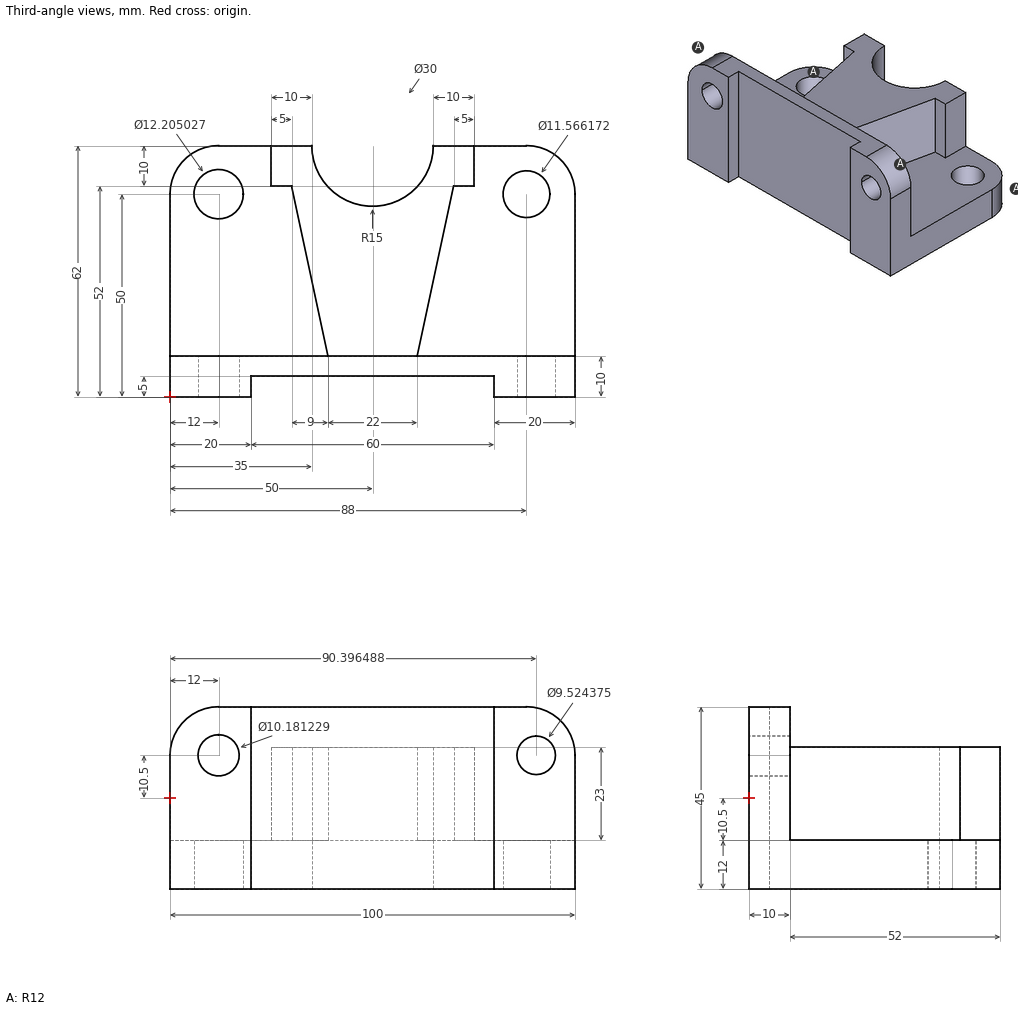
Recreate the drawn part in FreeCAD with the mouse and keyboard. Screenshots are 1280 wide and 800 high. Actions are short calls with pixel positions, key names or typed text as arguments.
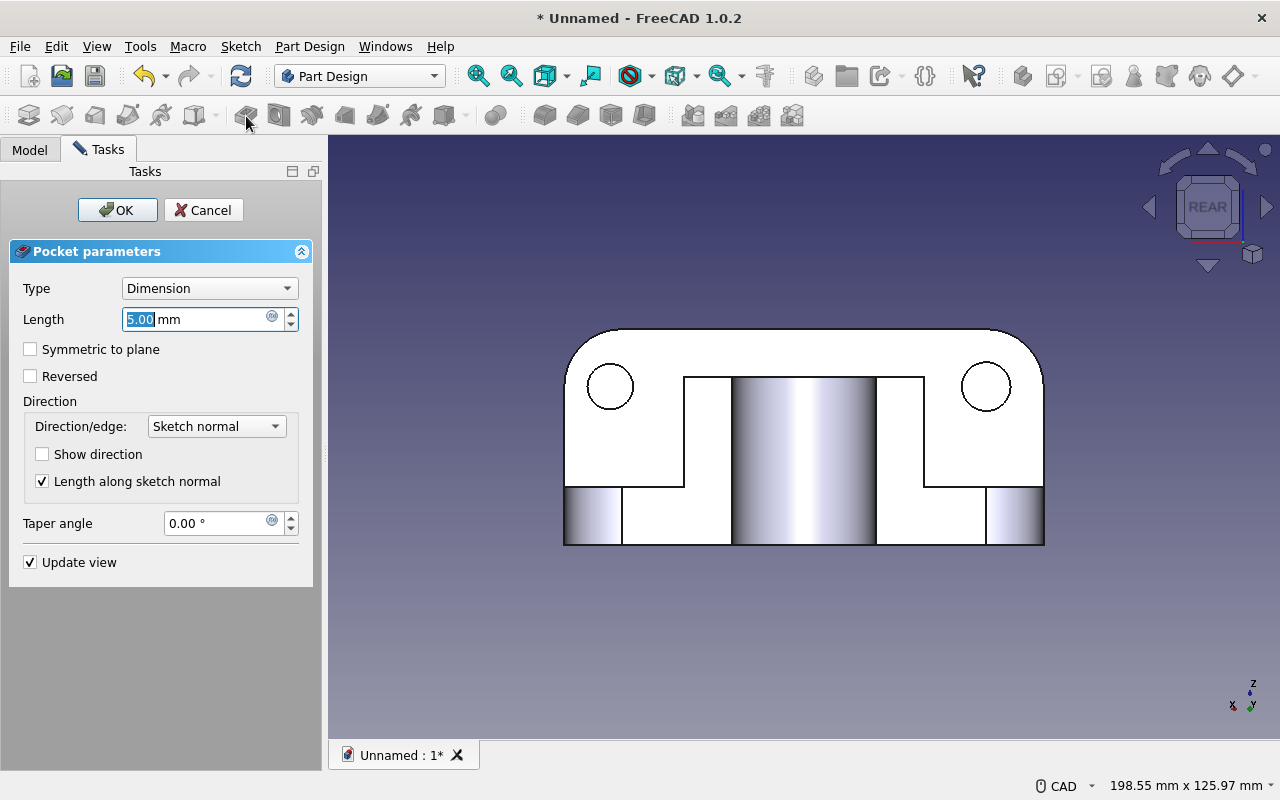
click(210, 288)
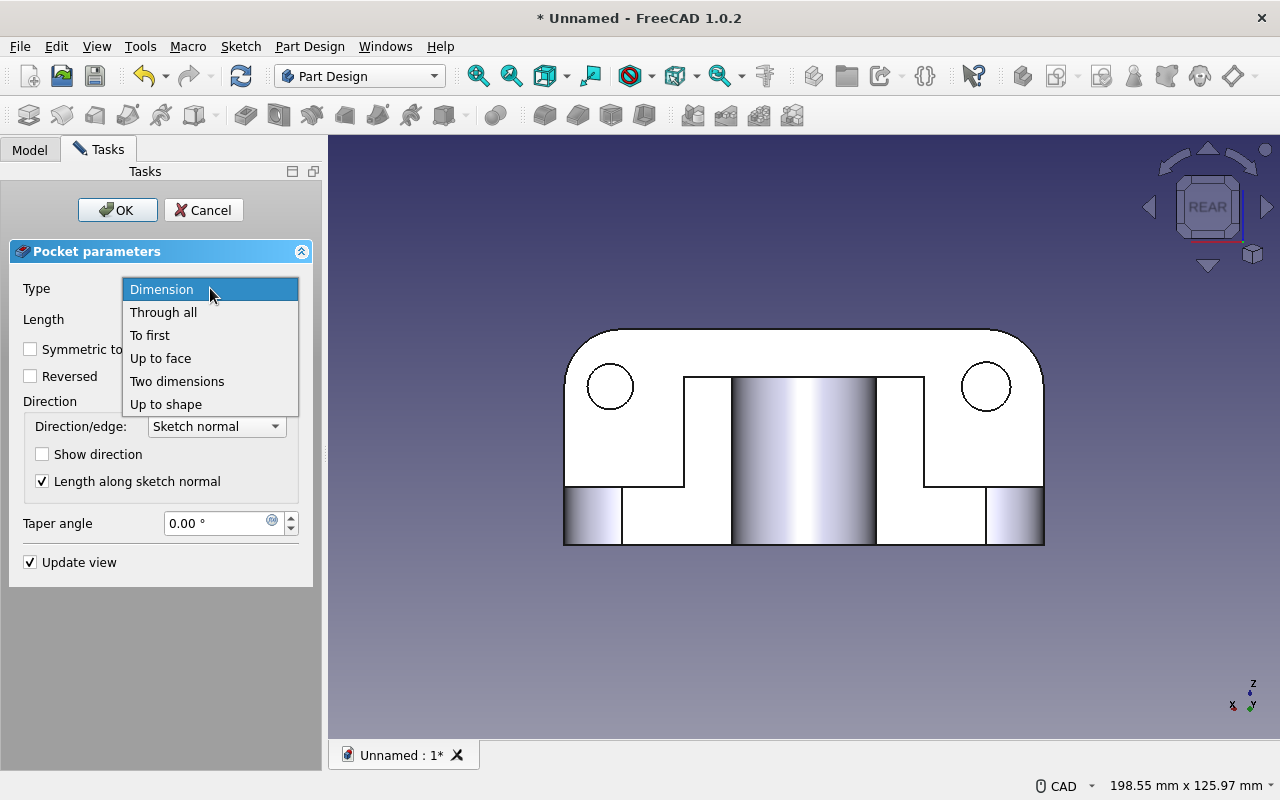
click(208, 312)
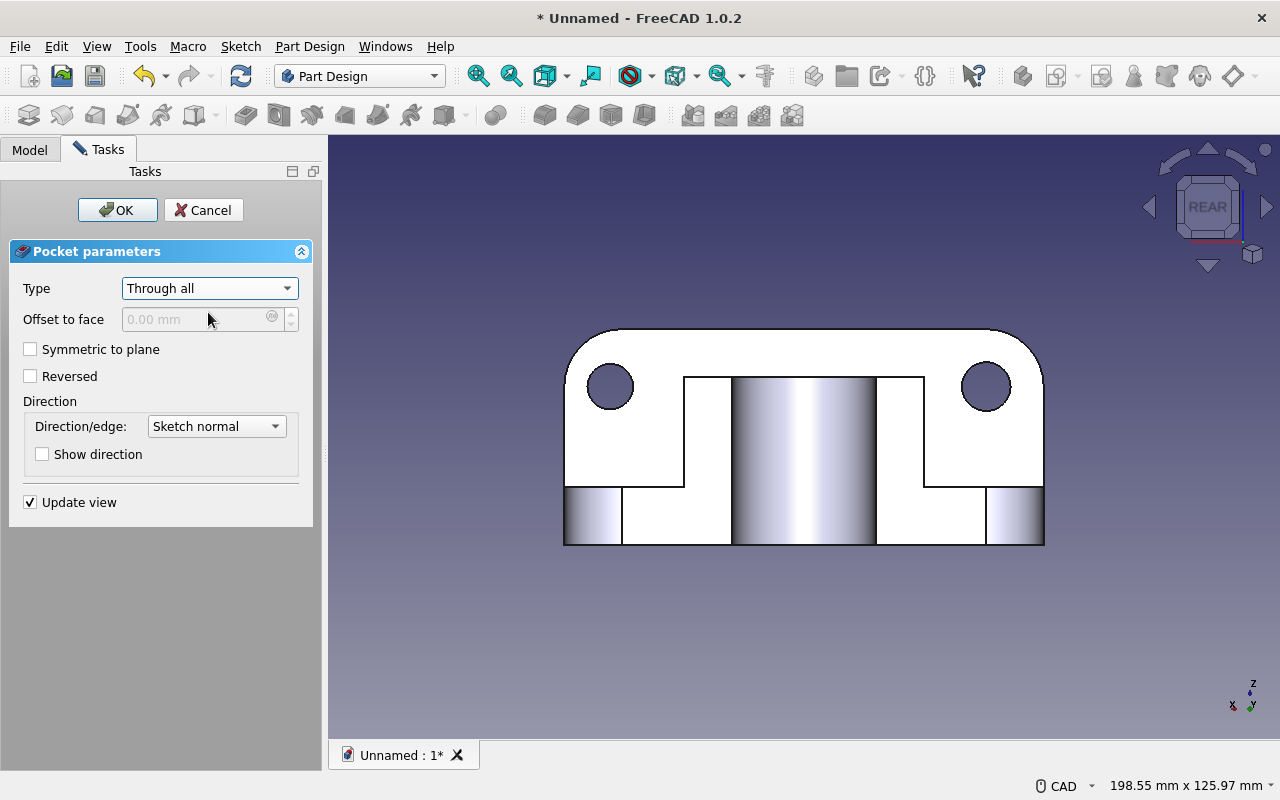
click(118, 210)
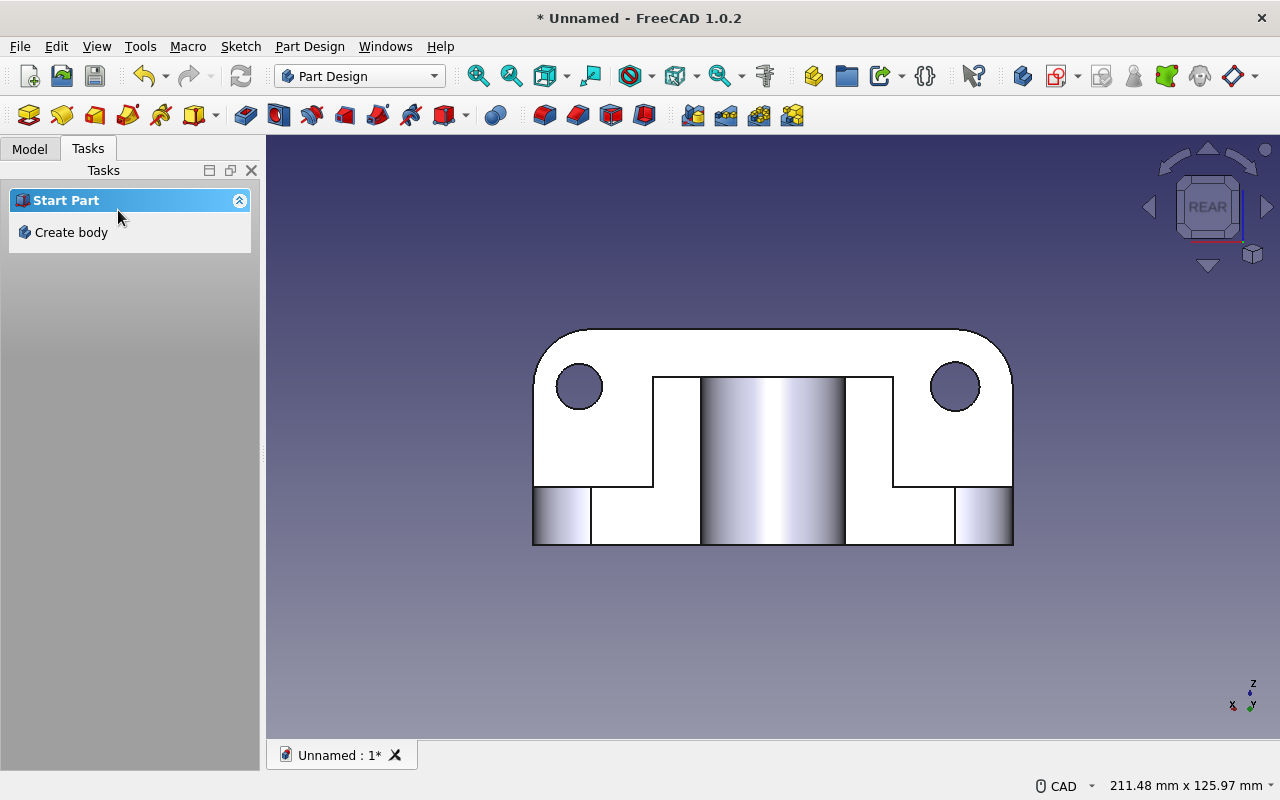
key(0)